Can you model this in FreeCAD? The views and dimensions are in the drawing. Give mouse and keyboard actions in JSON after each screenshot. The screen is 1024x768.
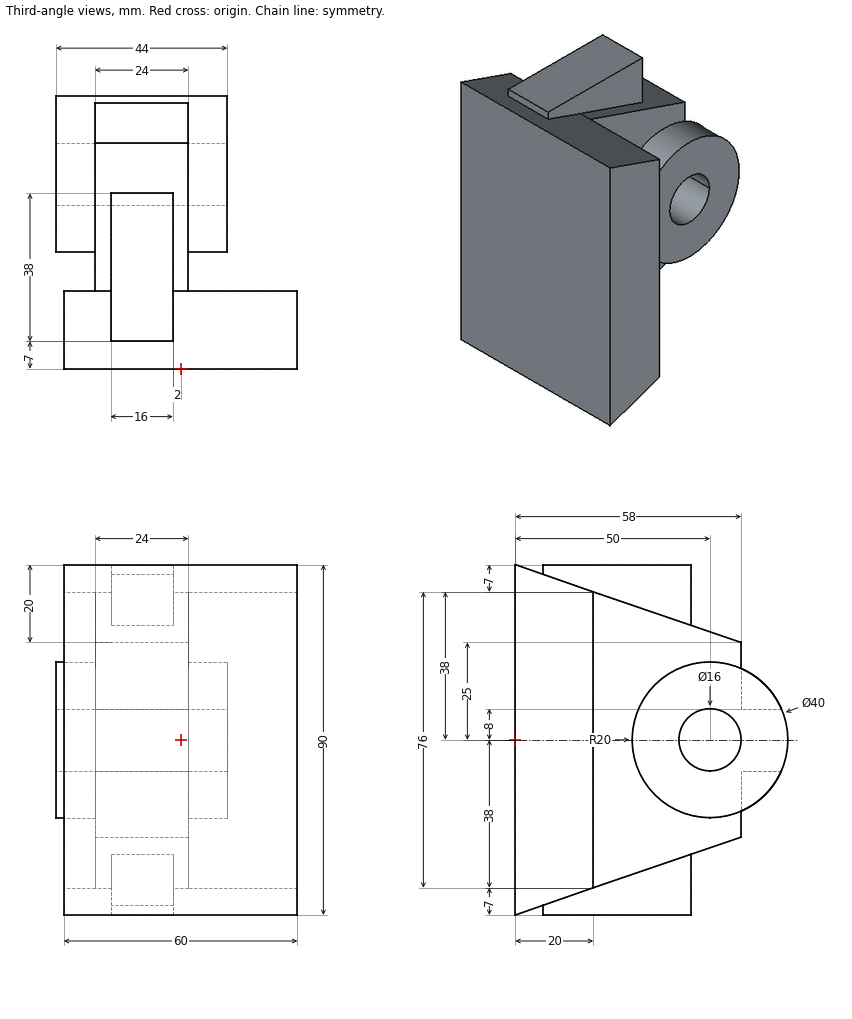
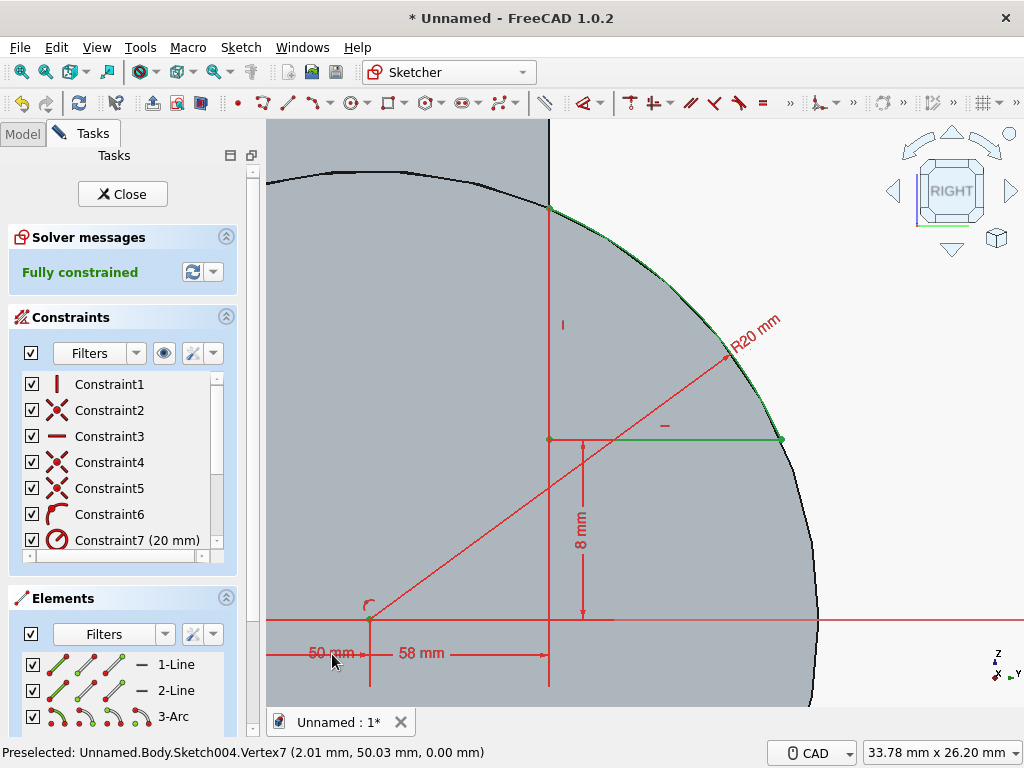
{"action": "left_click", "coordinate": [123, 194]}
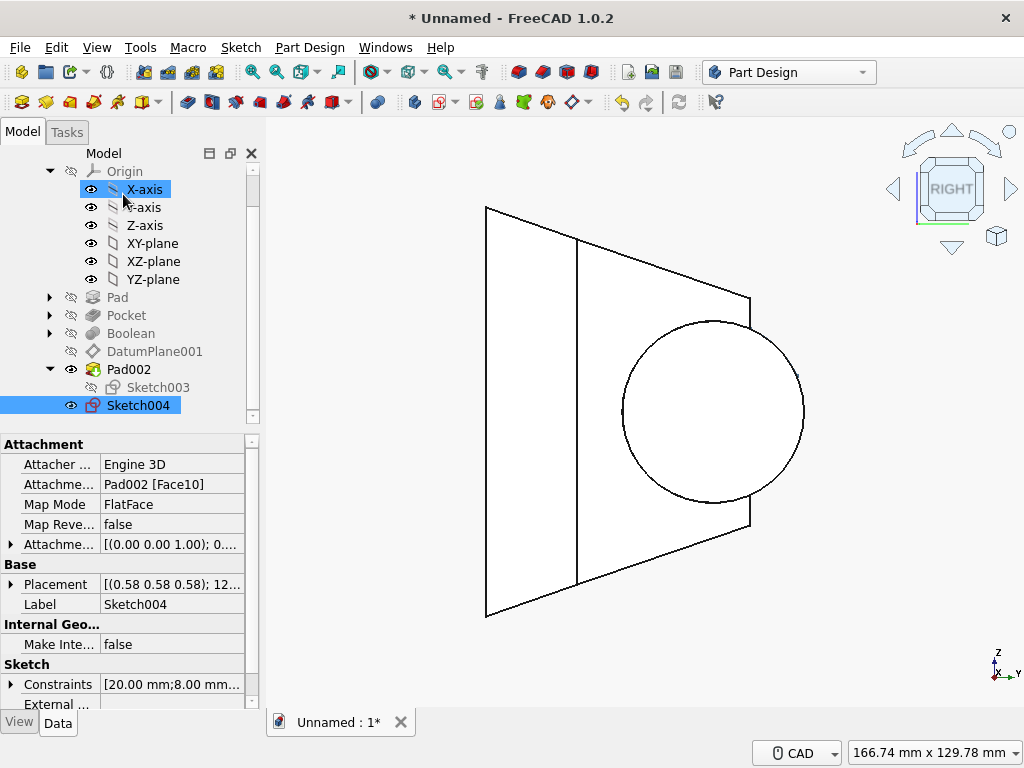
{"action": "left_click", "coordinate": [188, 102]}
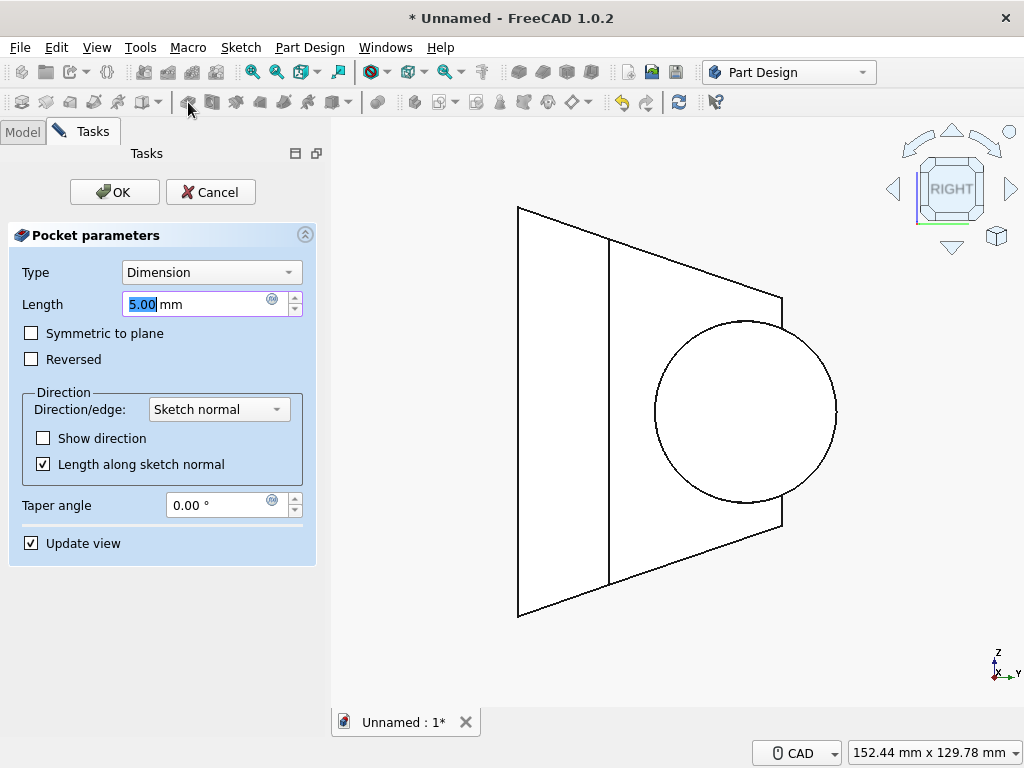
{"action": "type", "text": "24"}
{"action": "key", "text": "Tab"}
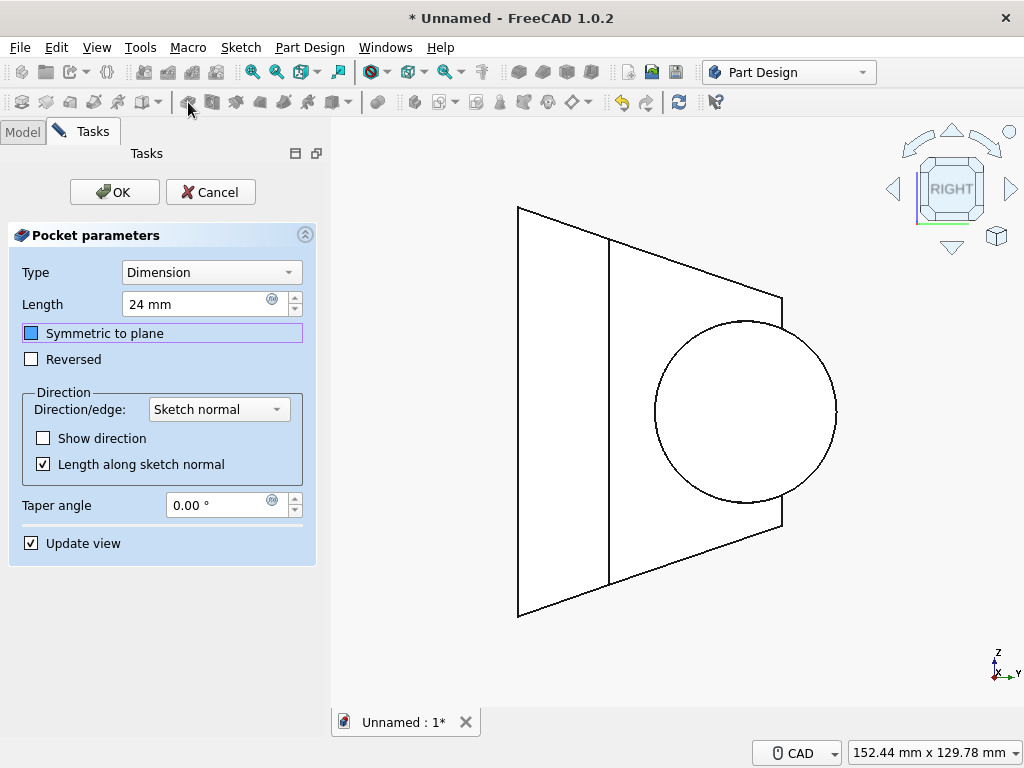
{"action": "left_click", "coordinate": [115, 192]}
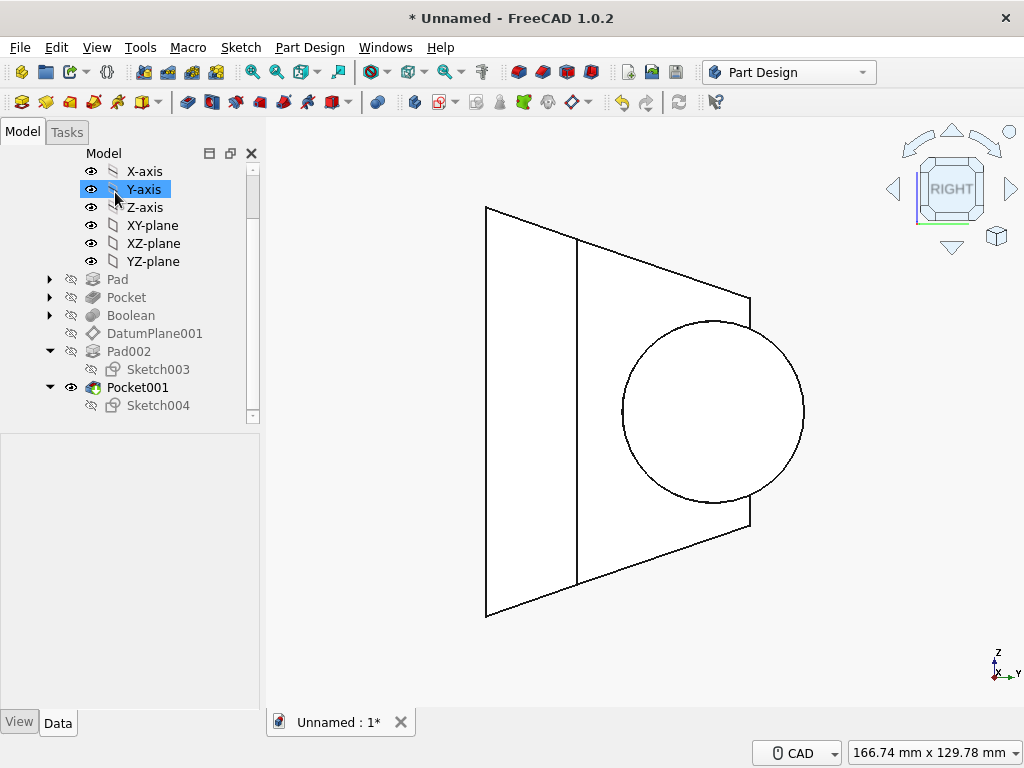
{"action": "left_click", "coordinate": [116, 387]}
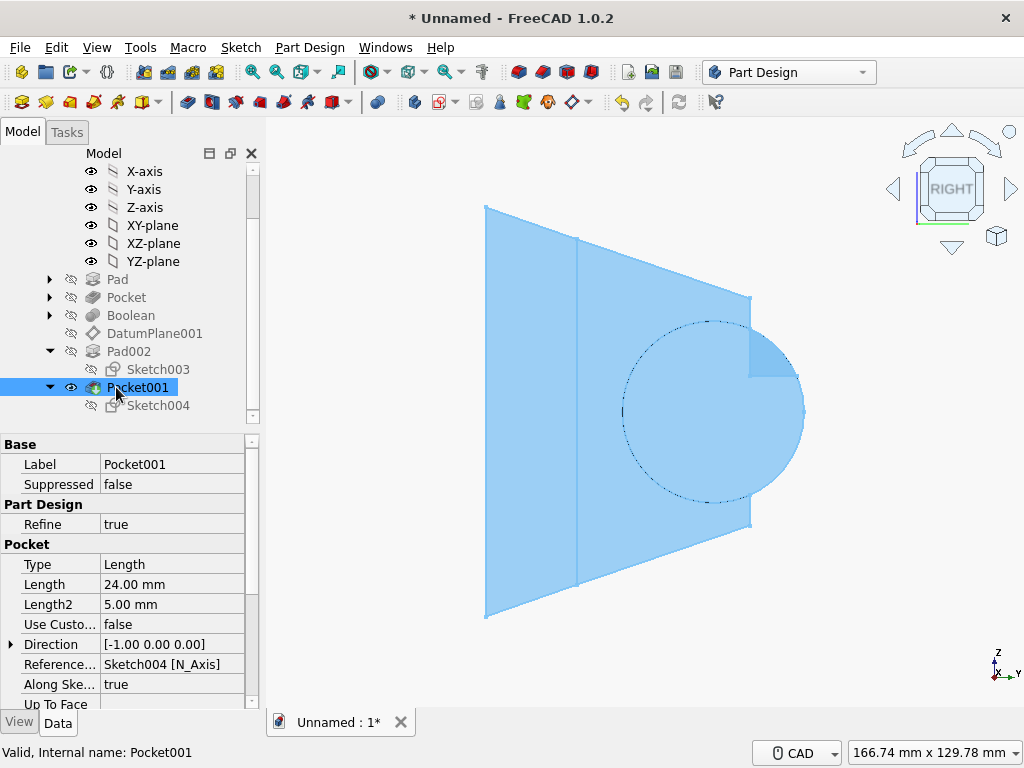
{"action": "left_click", "coordinate": [144, 72]}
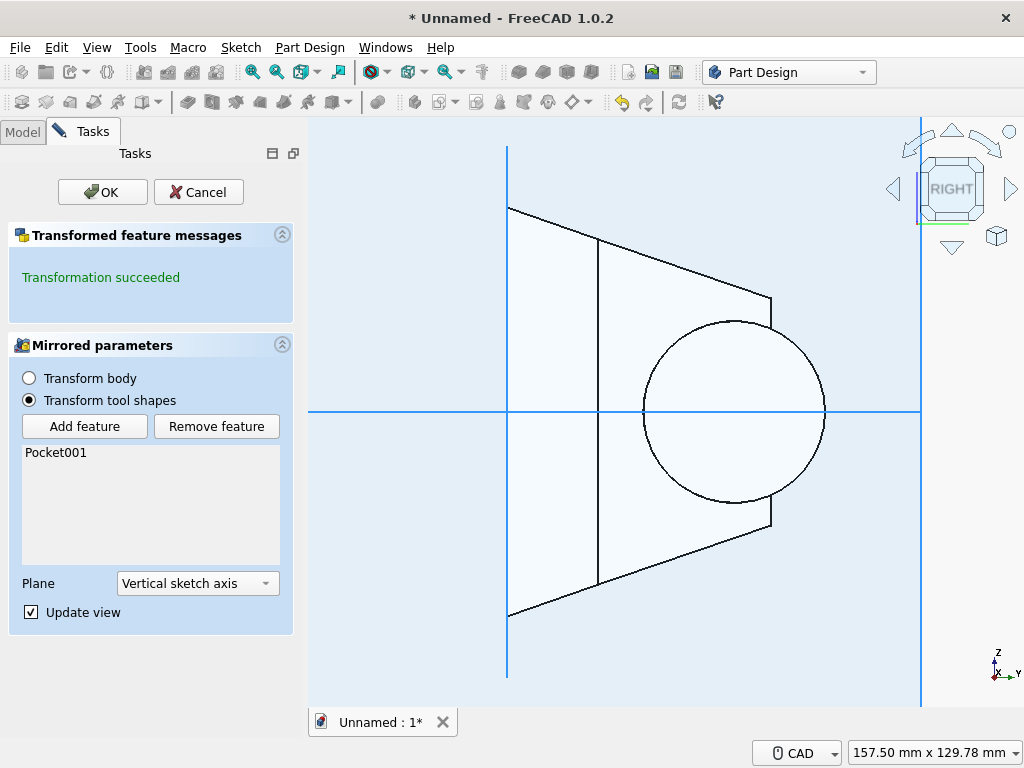
{"action": "left_click", "coordinate": [198, 584]}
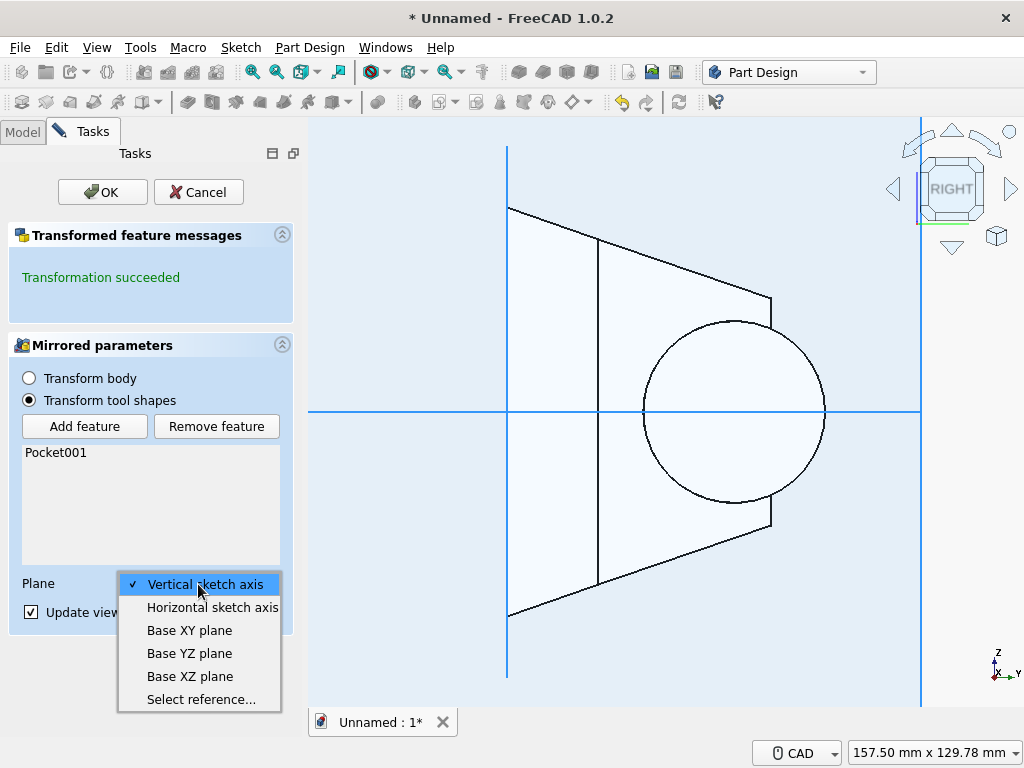
{"action": "left_click", "coordinate": [198, 630]}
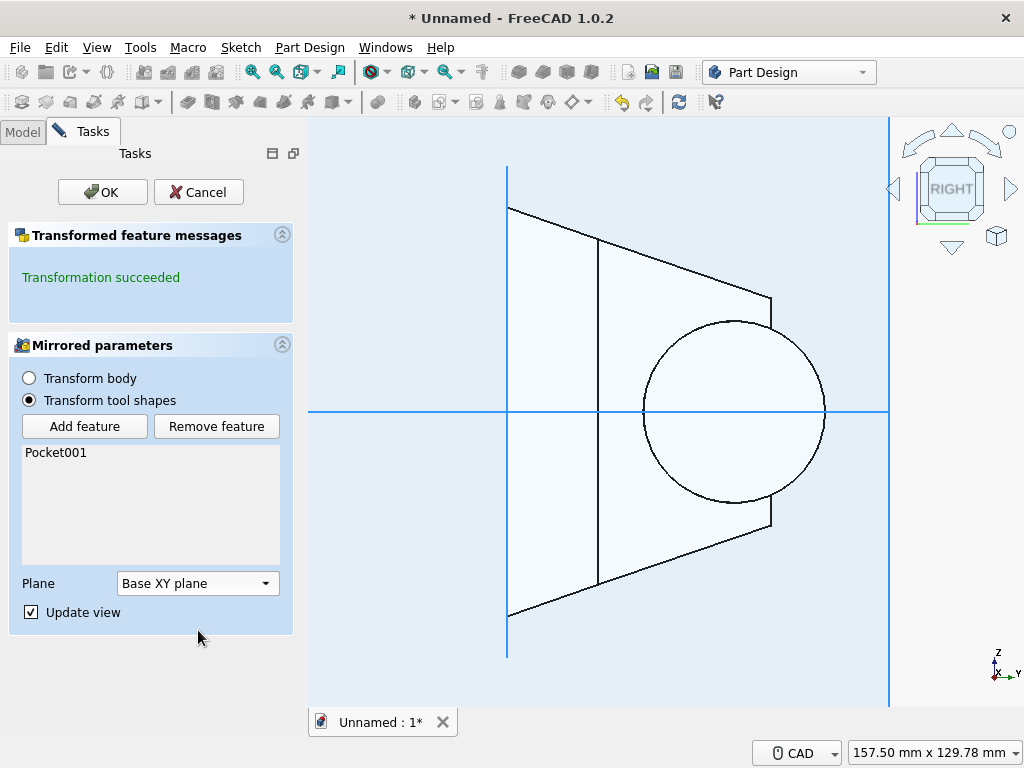
{"action": "left_click", "coordinate": [103, 192]}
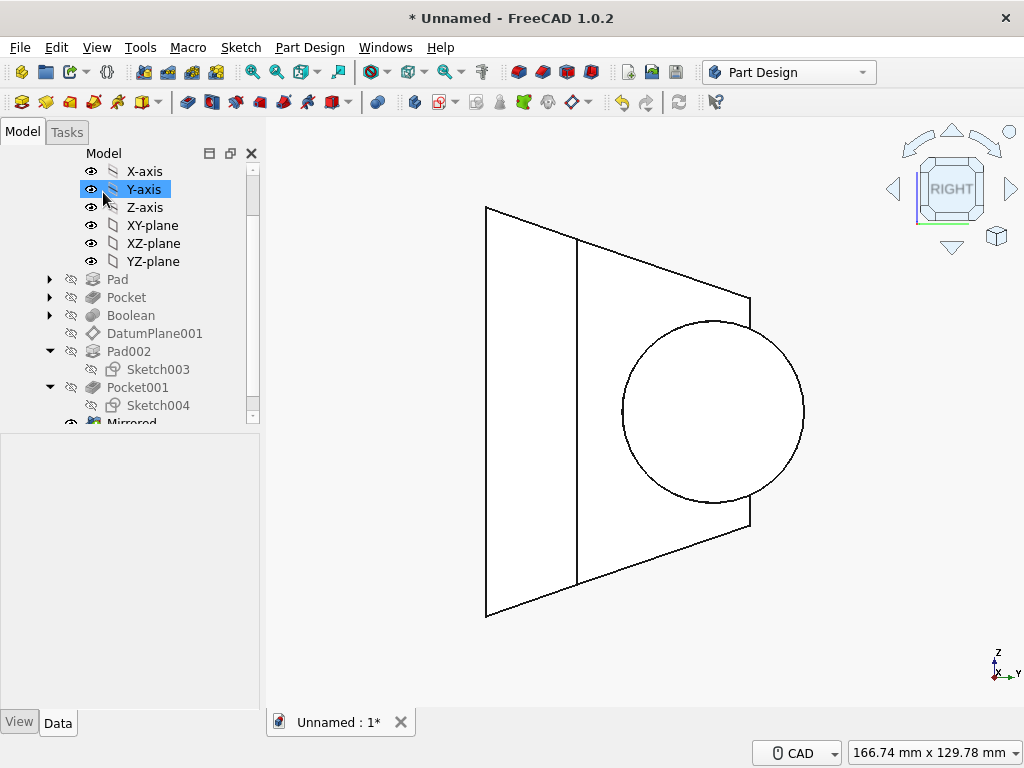
{"action": "left_click", "coordinate": [713, 411]}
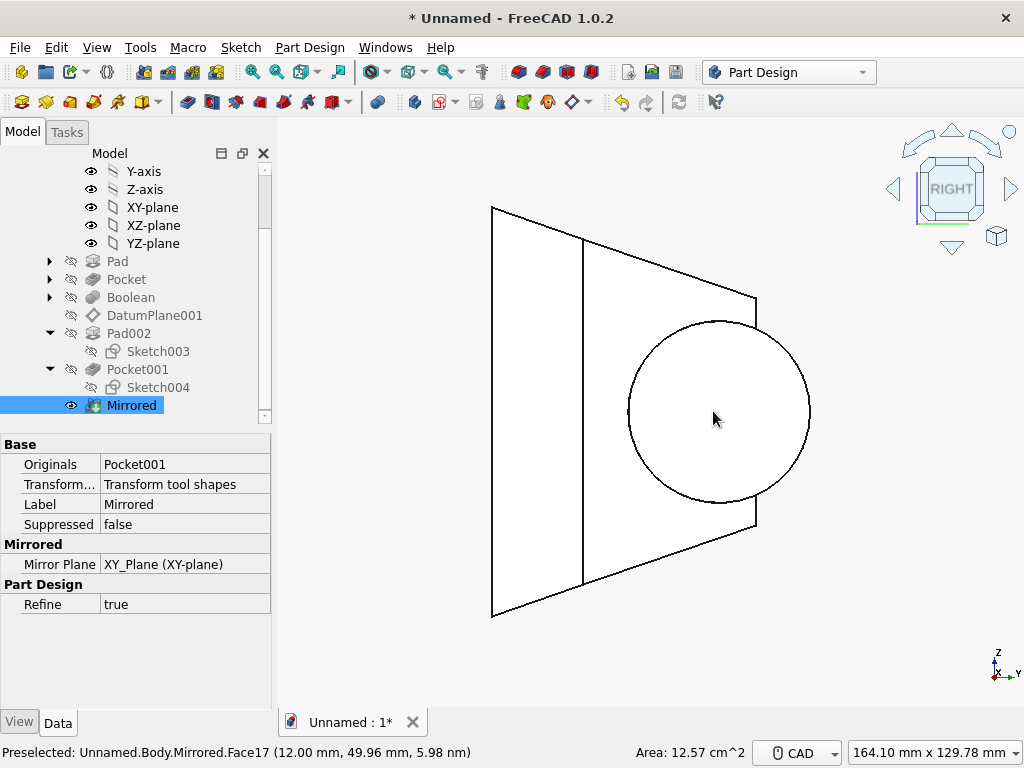
{"action": "left_click", "coordinate": [440, 102]}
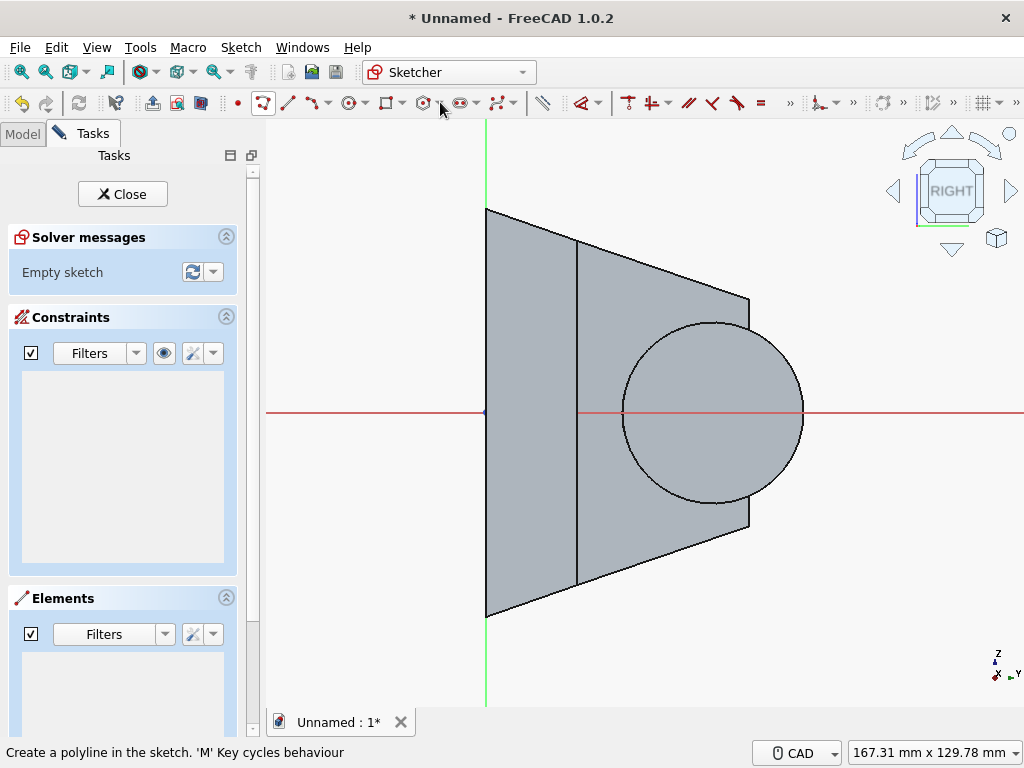
{"action": "scroll", "coordinate": [747, 413], "scroll_direction": "up", "scroll_amount": 8}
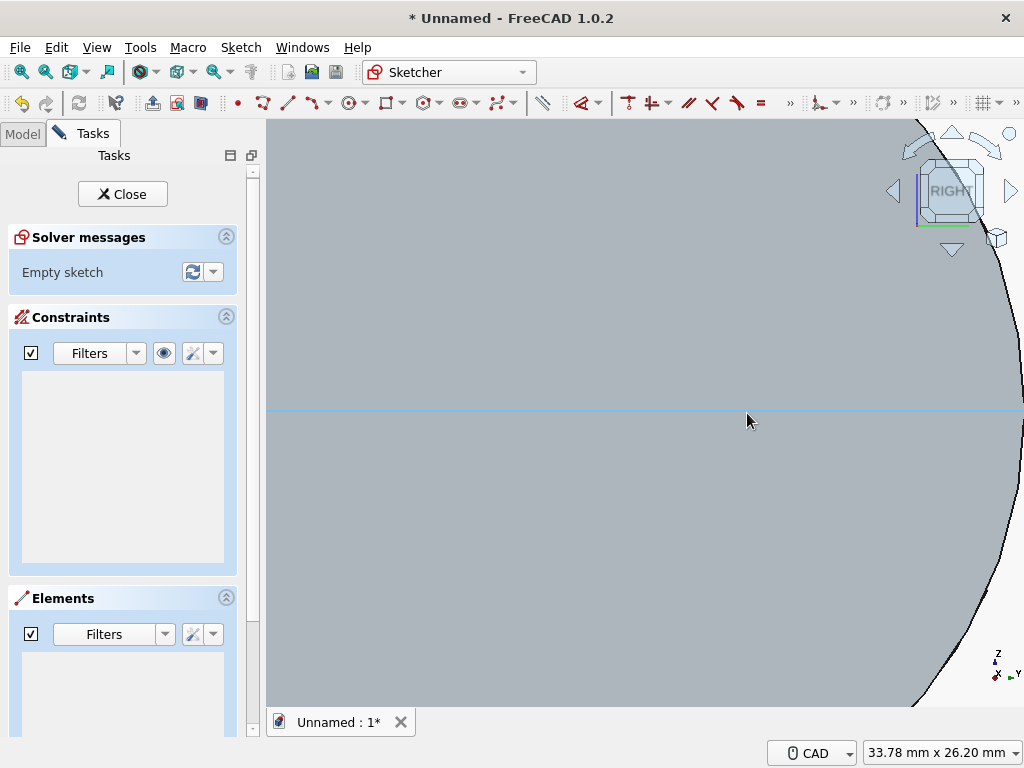
{"action": "left_click", "coordinate": [350, 104]}